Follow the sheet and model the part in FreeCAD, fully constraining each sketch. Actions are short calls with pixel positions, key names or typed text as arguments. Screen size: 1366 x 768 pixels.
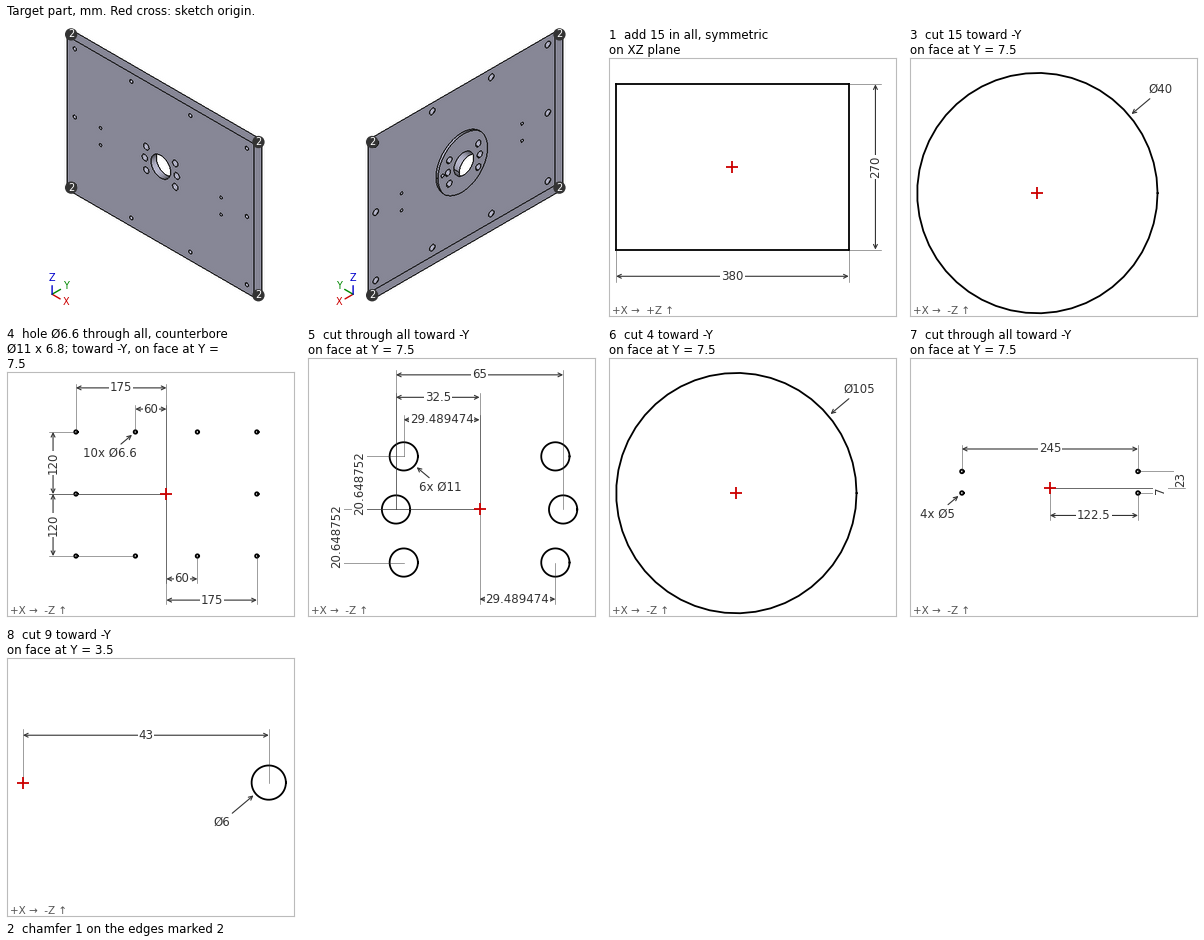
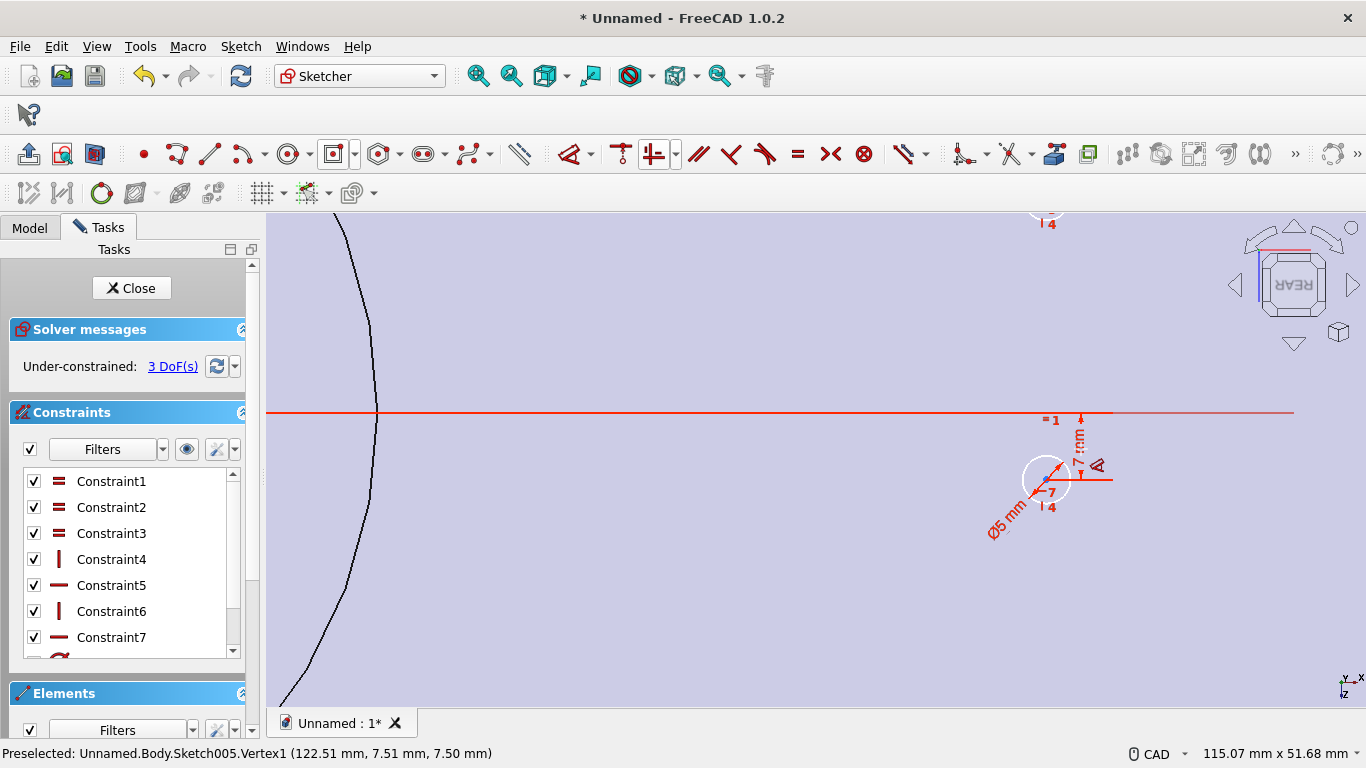
scroll(1033, 500, down, 7)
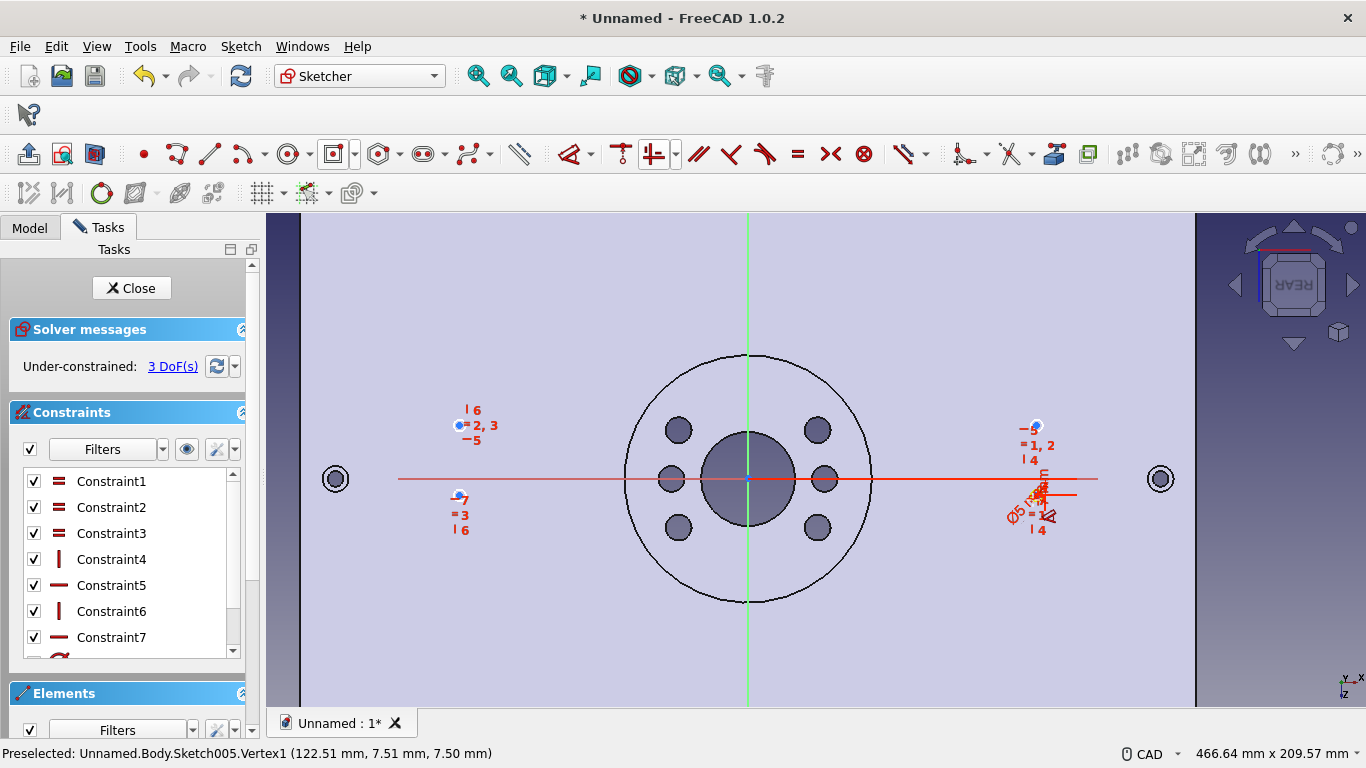
click(1037, 426)
click(1071, 452)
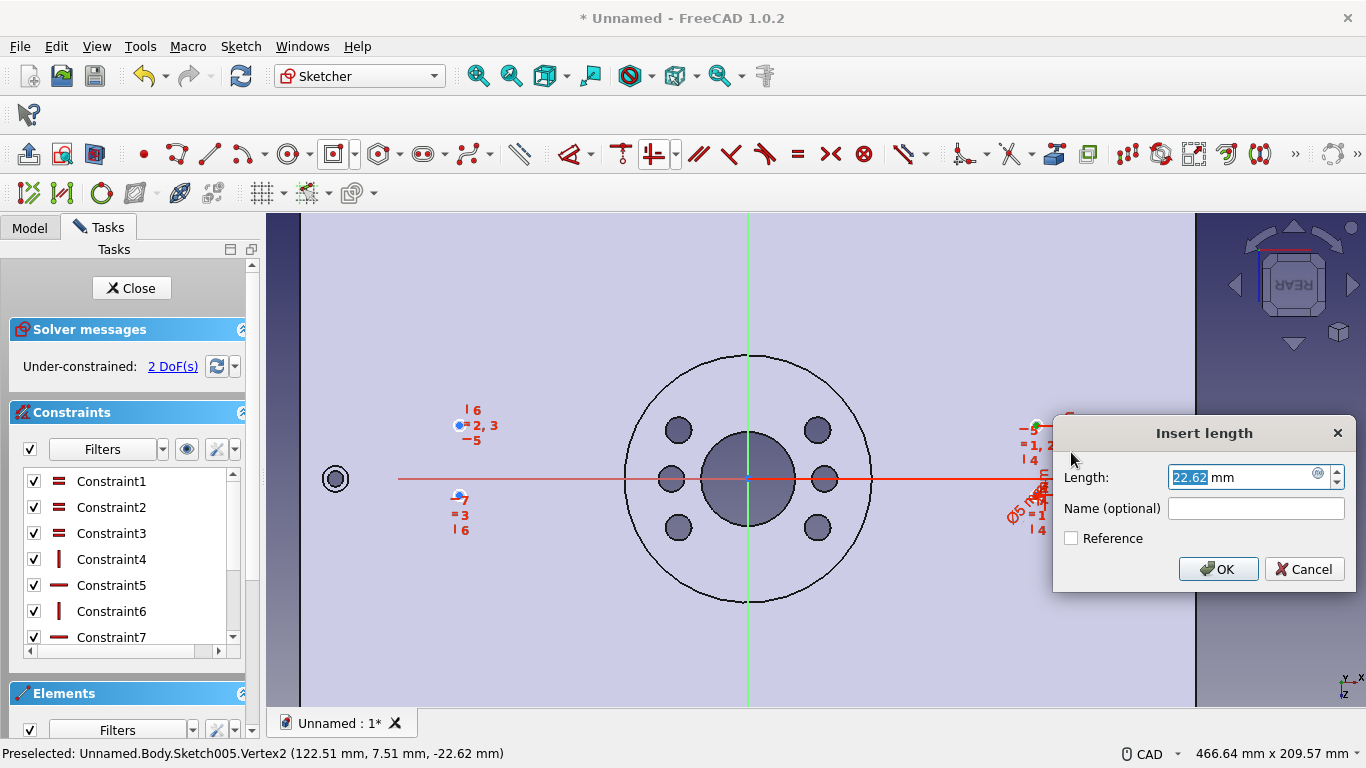
text(23)
key(Return)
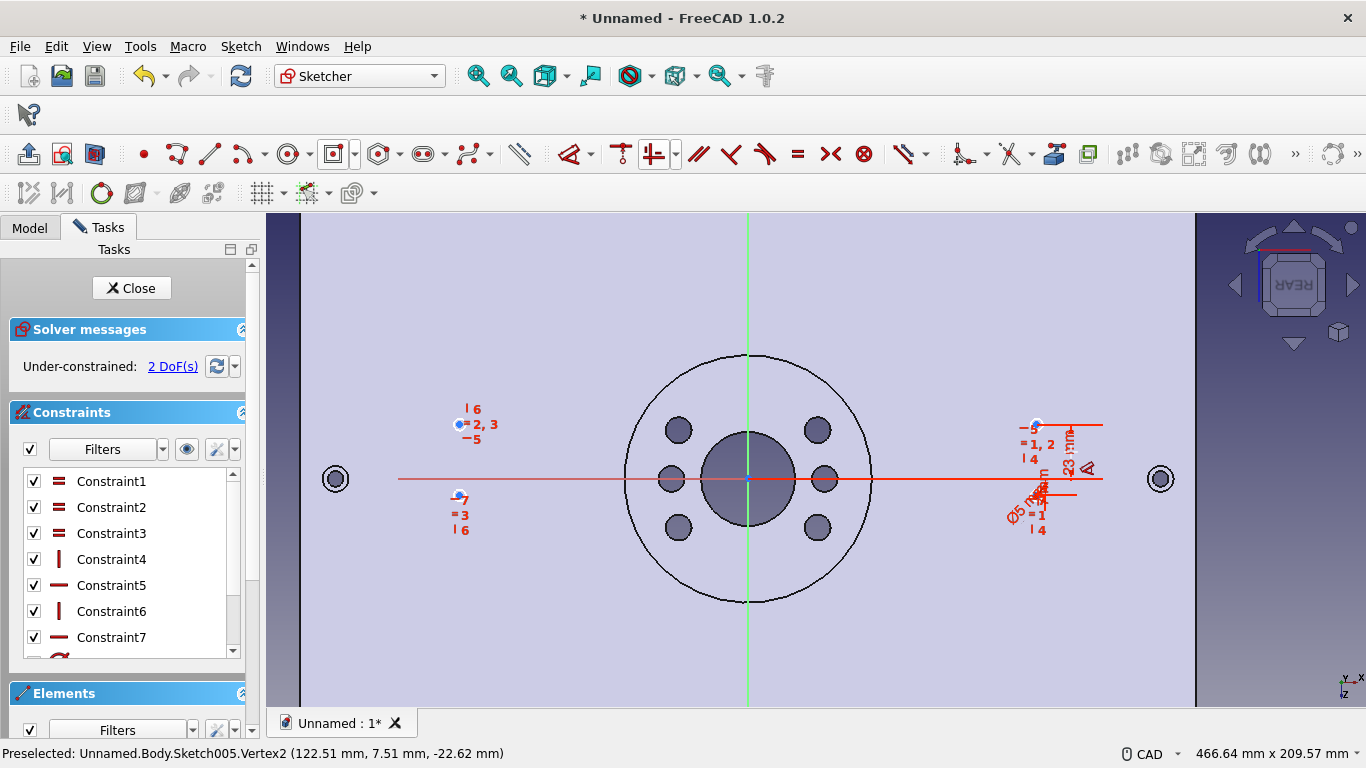
click(1037, 425)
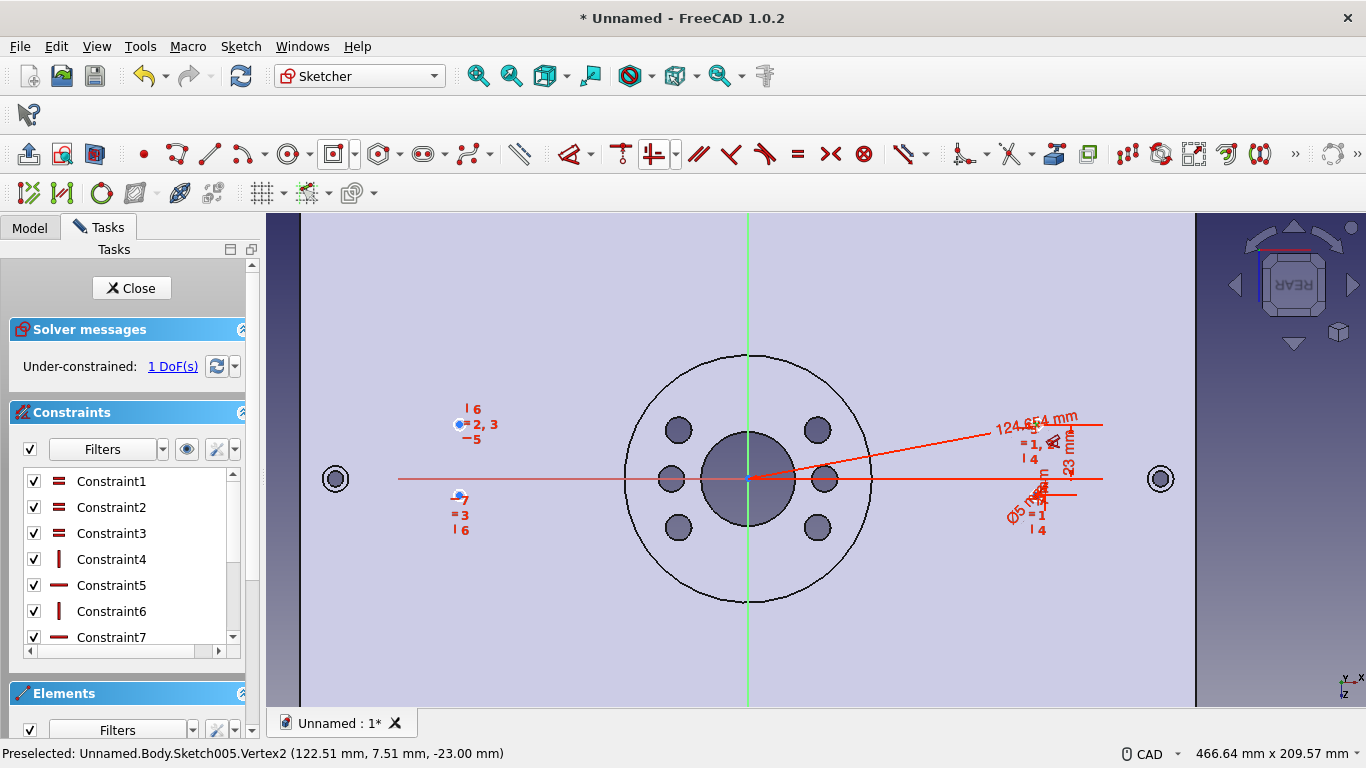
click(460, 425)
click(616, 391)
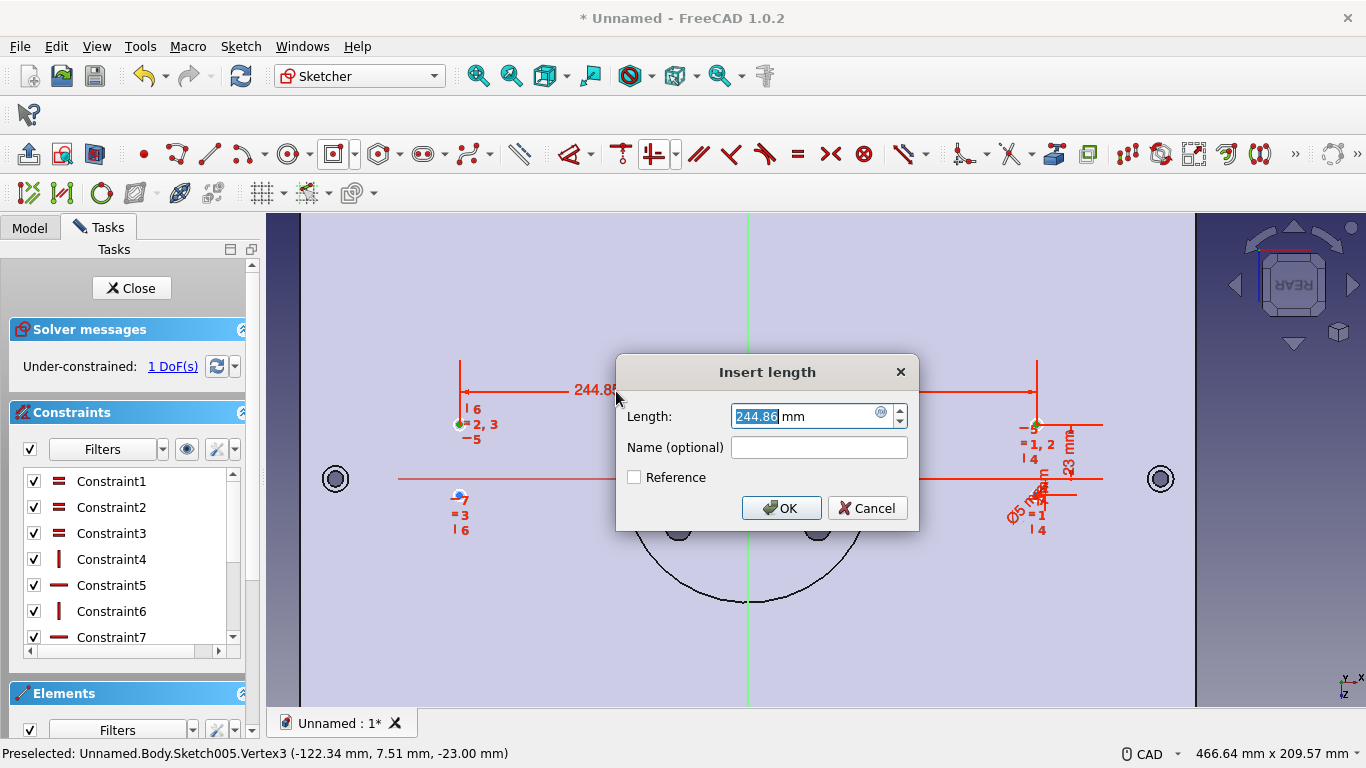
text(245)
key(Return)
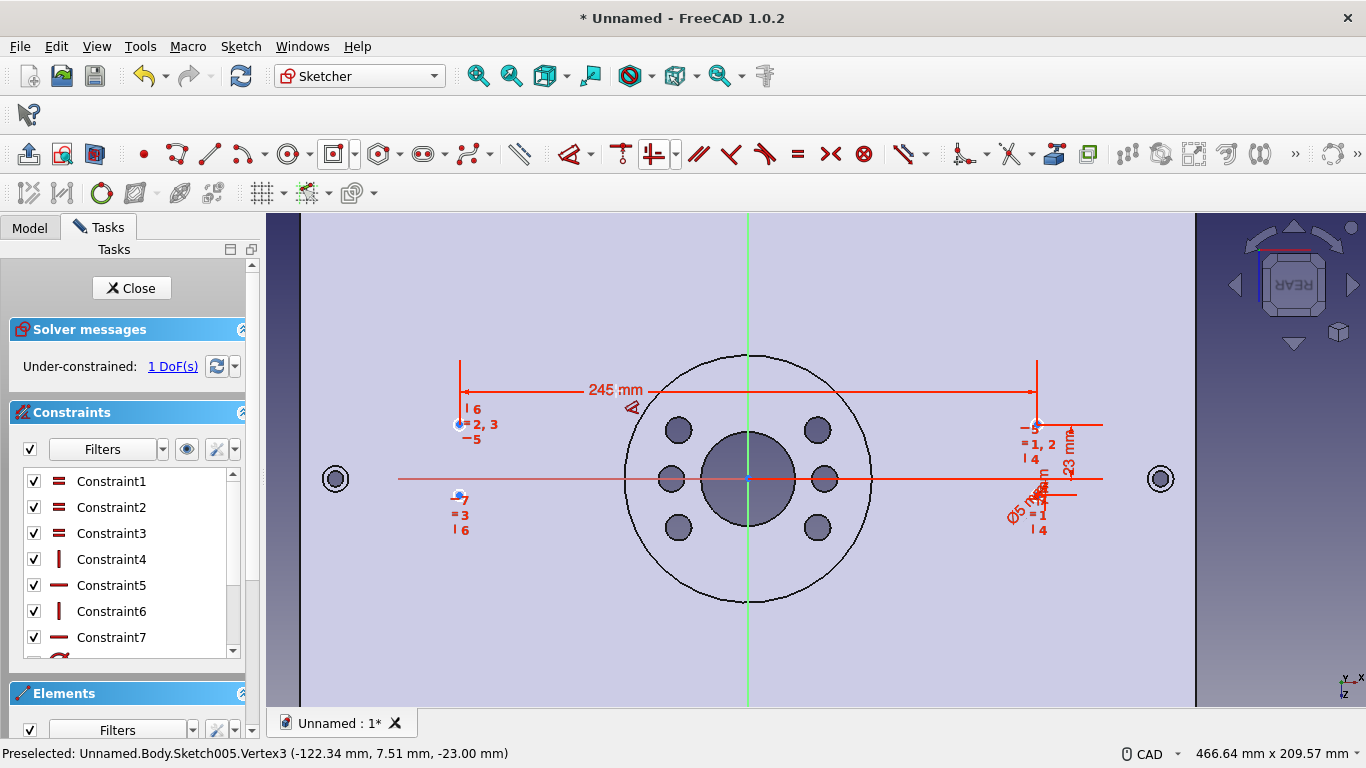
click(1037, 495)
click(893, 529)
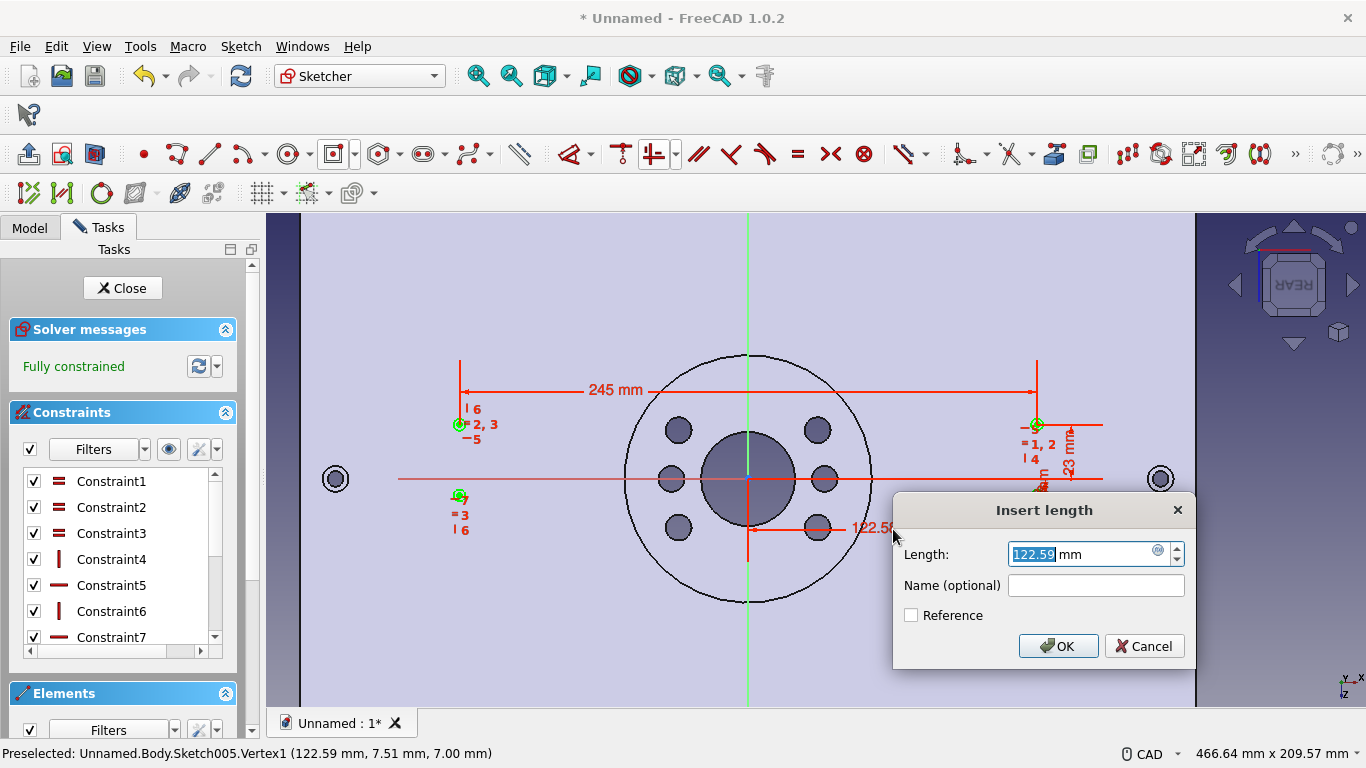
text(122.5)
key(Return)
key(Escape)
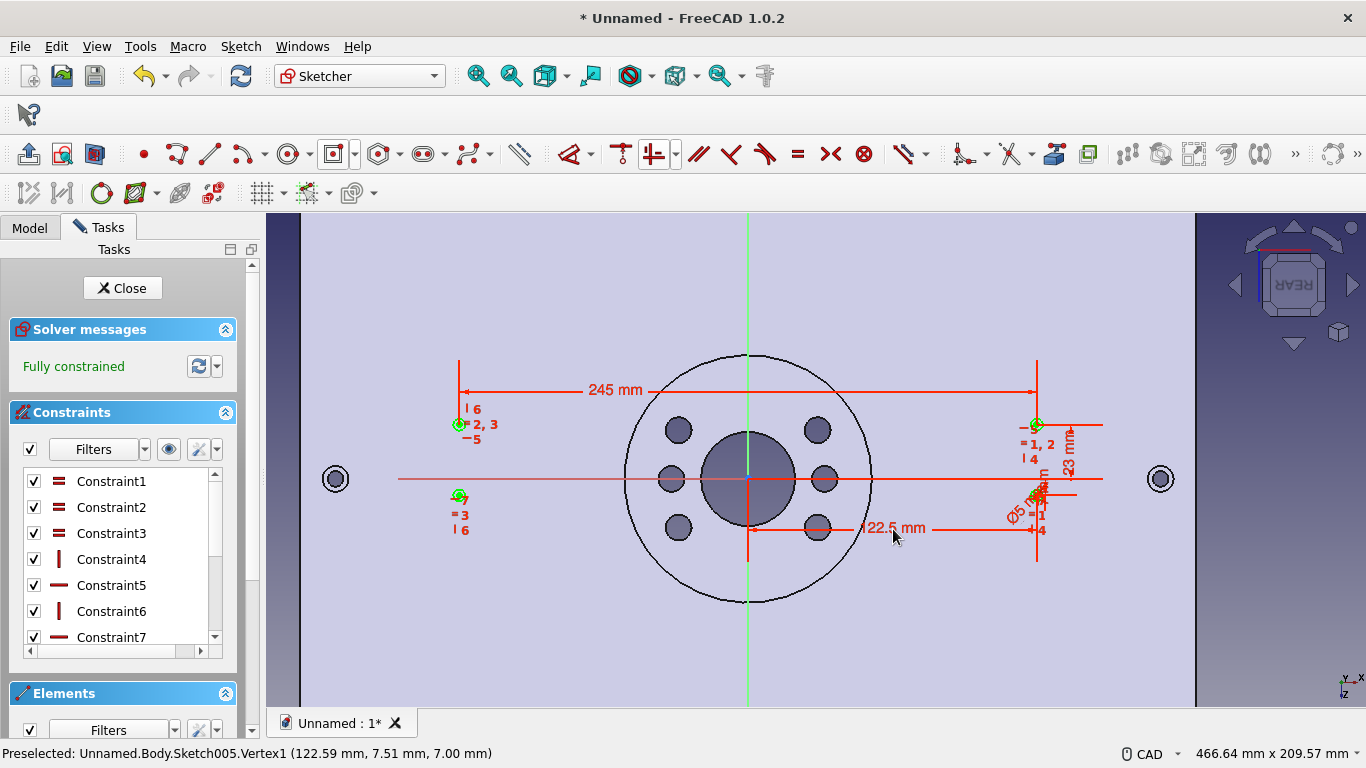
click(123, 288)